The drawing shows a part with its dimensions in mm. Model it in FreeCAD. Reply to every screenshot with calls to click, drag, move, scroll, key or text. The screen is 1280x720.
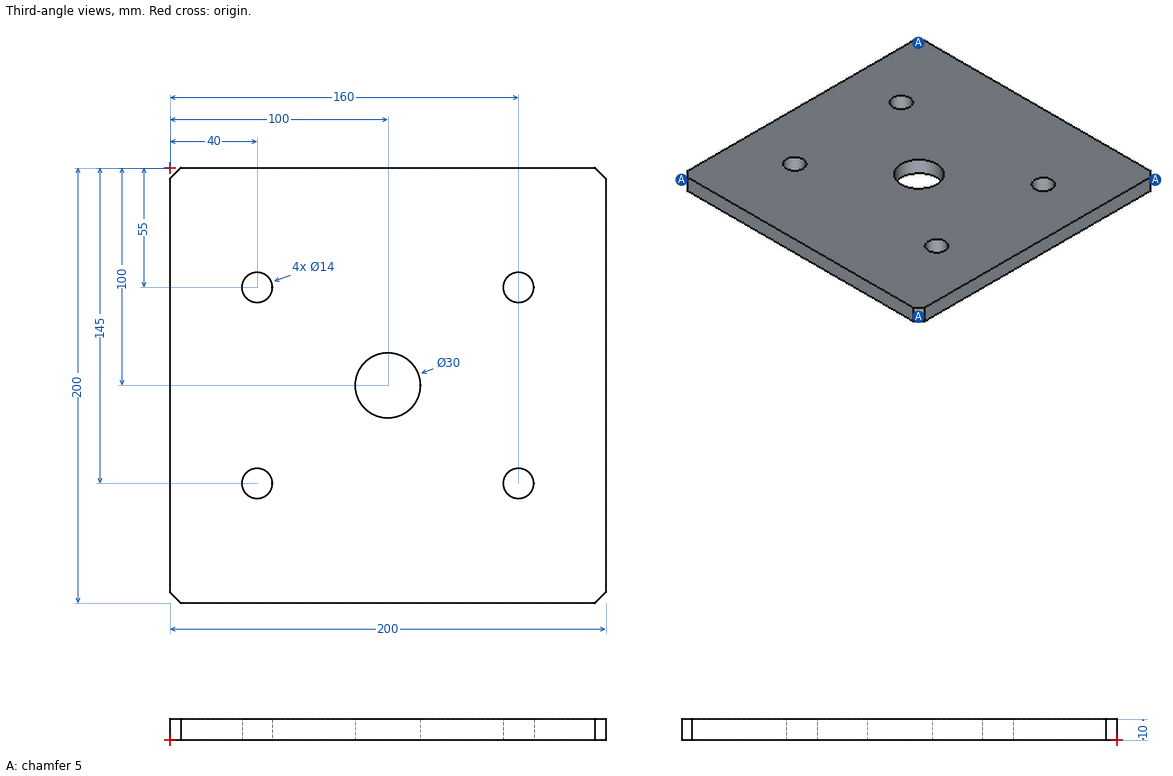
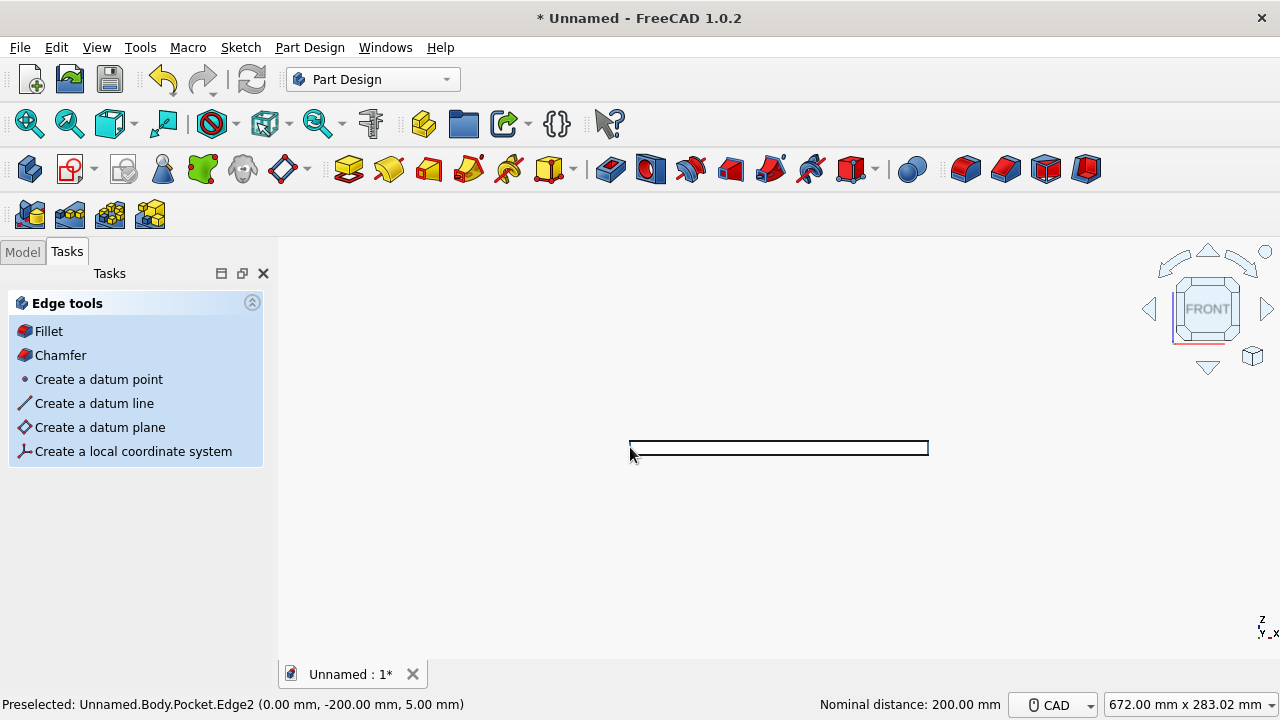
scroll(630, 447, up, 5)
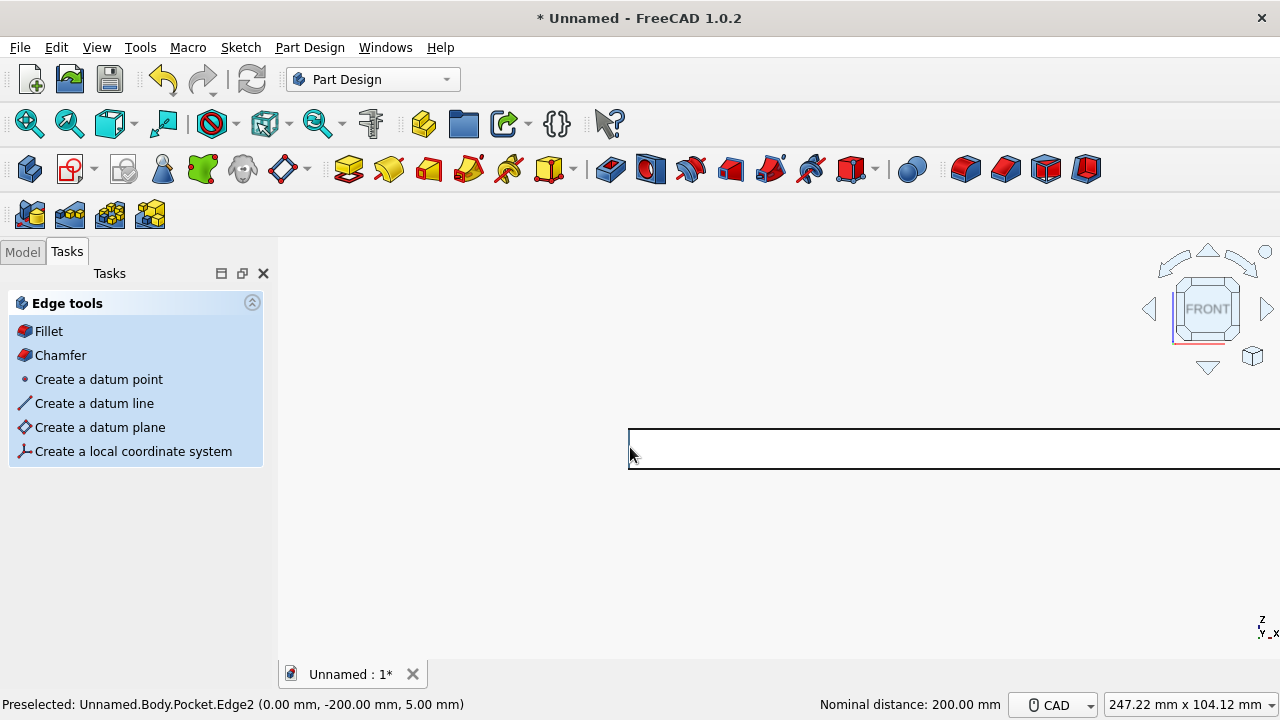
click(30, 124)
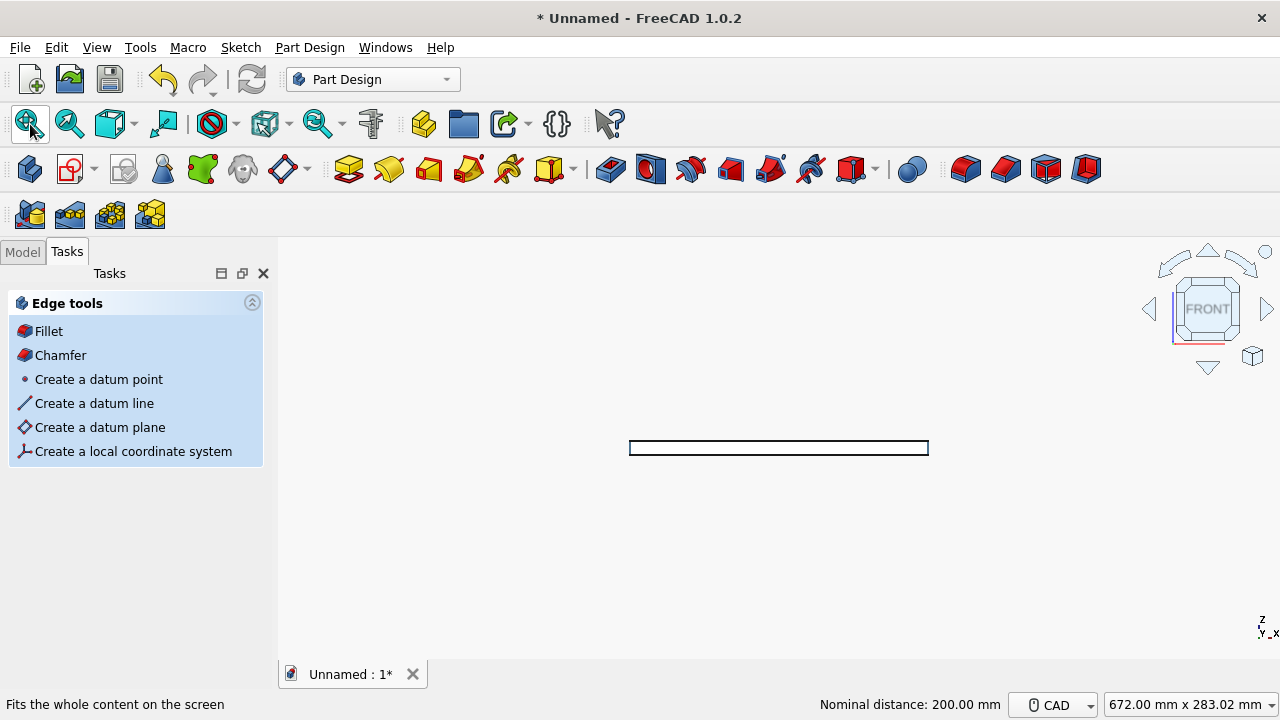
key(3)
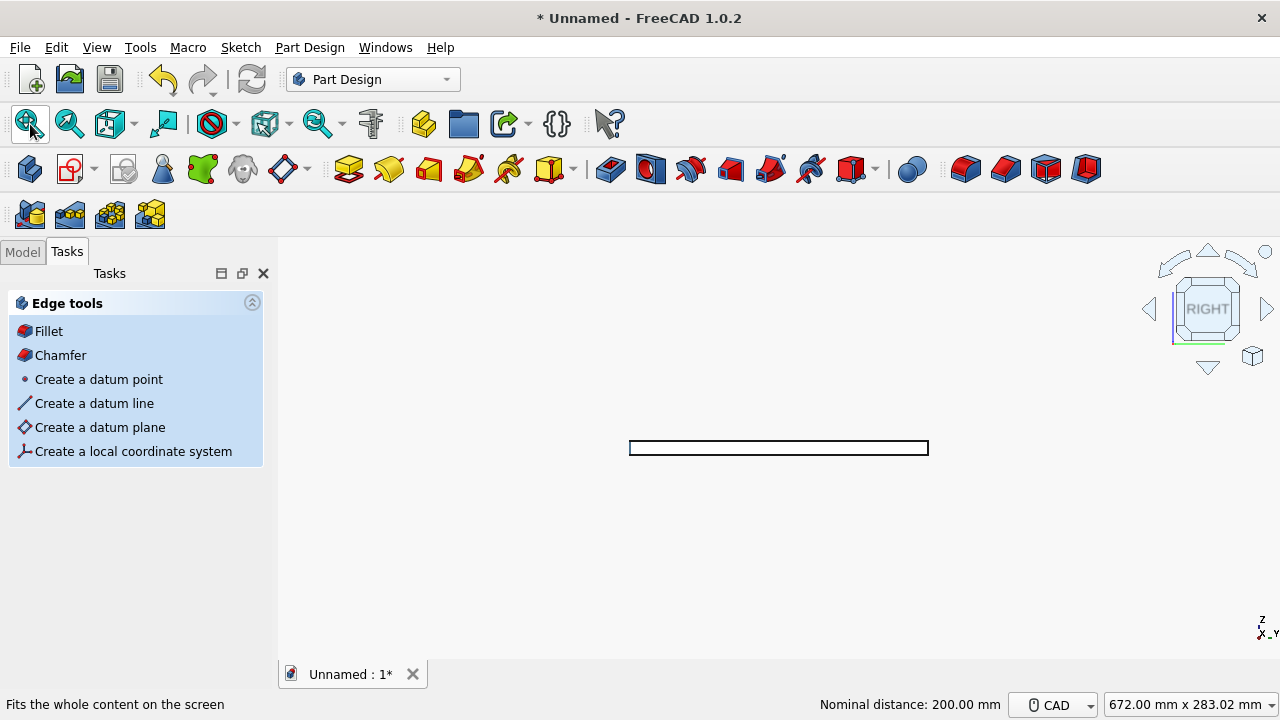
click(30, 124)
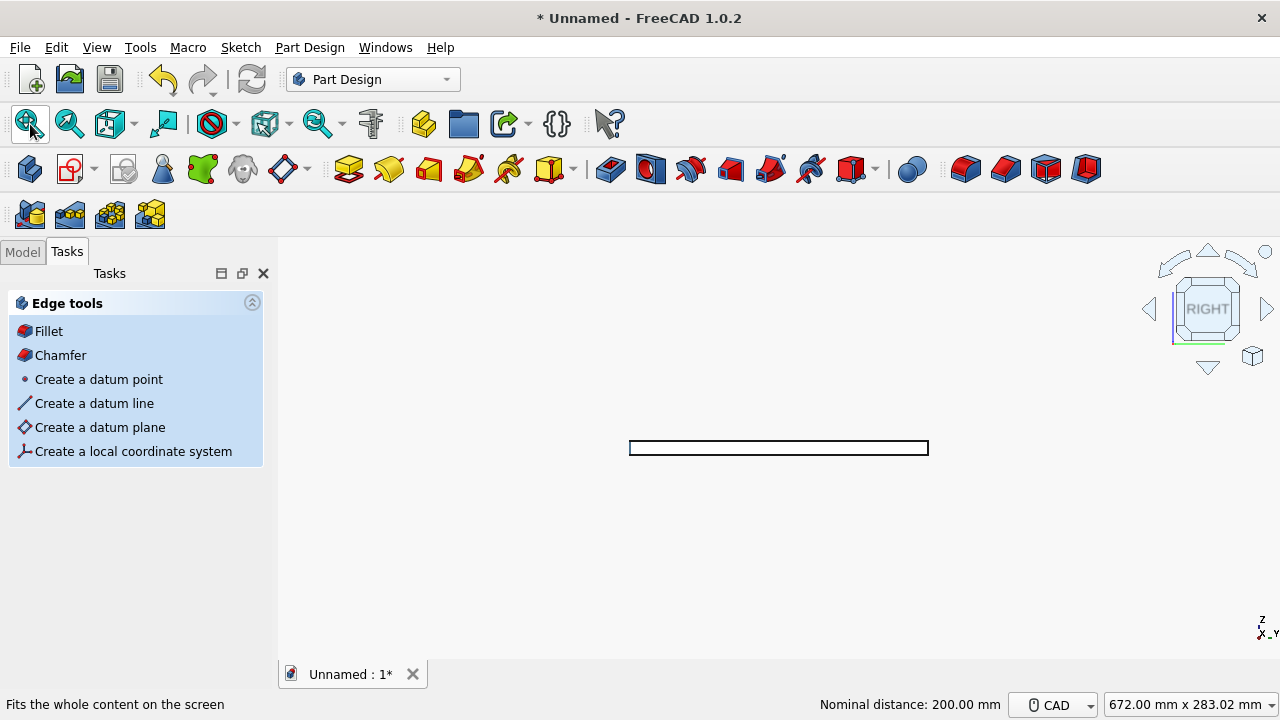
click(928, 447, ctrl)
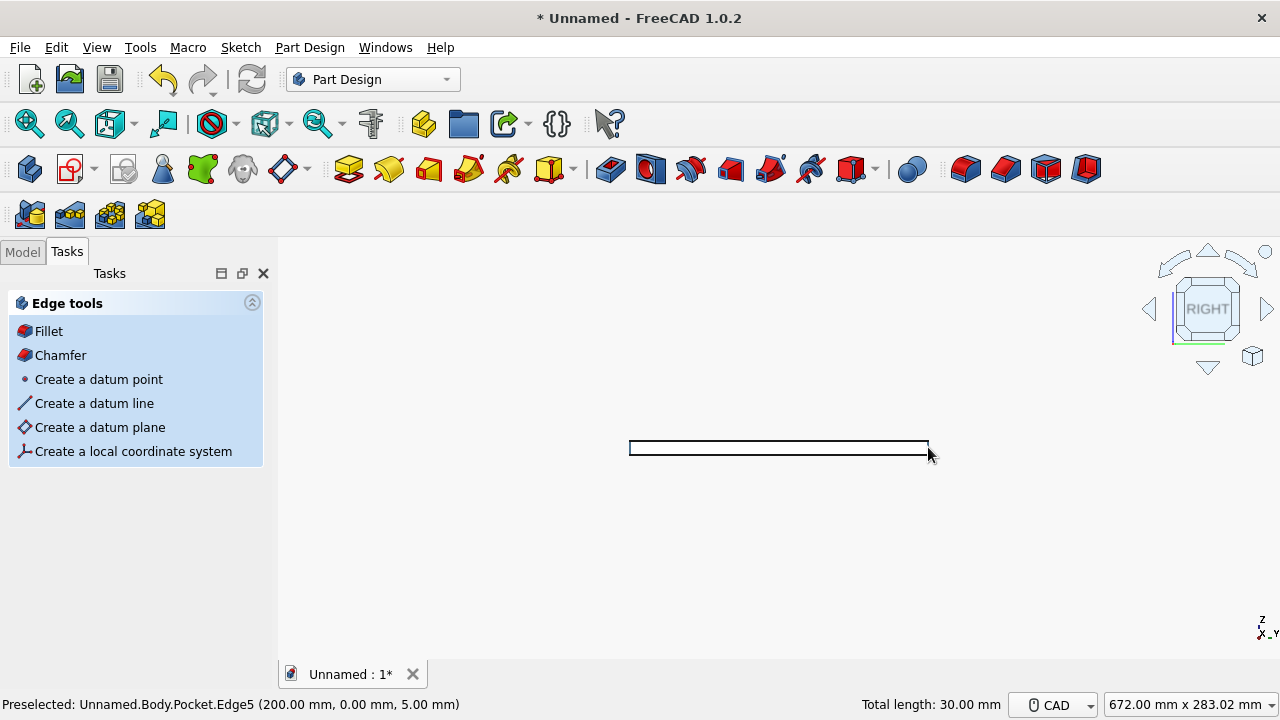
scroll(928, 447, up, 5)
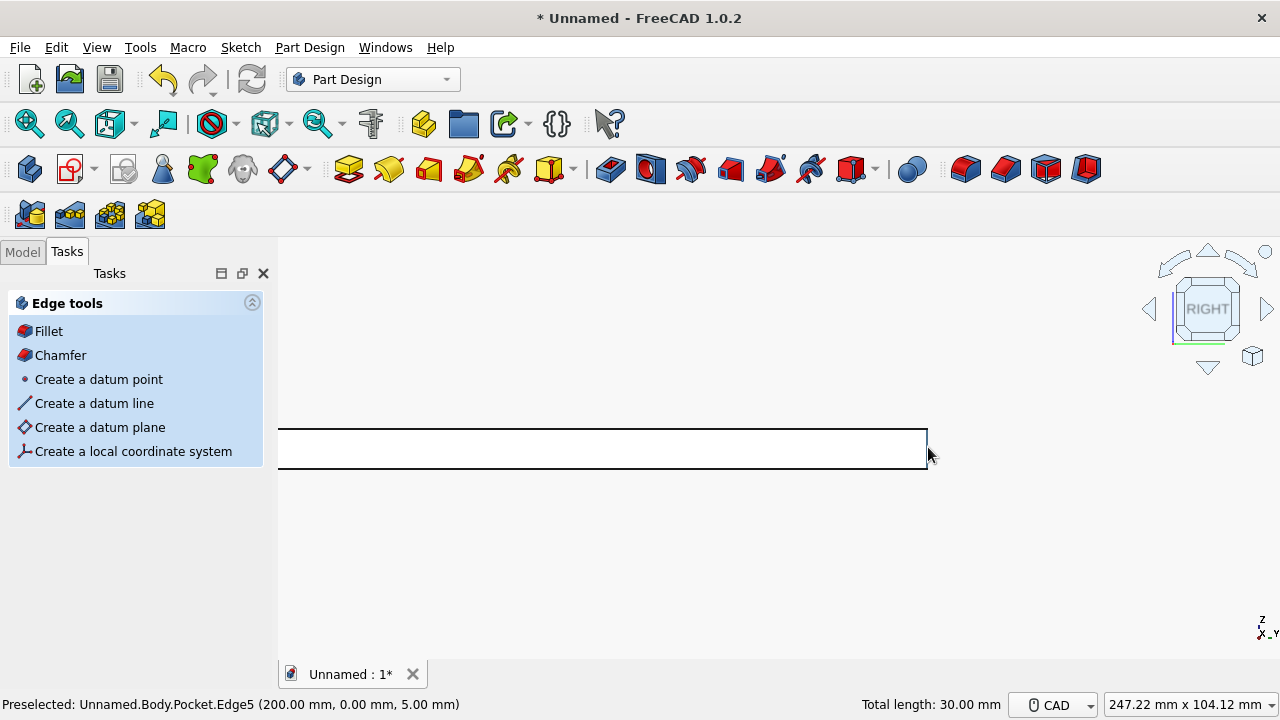
click(30, 124)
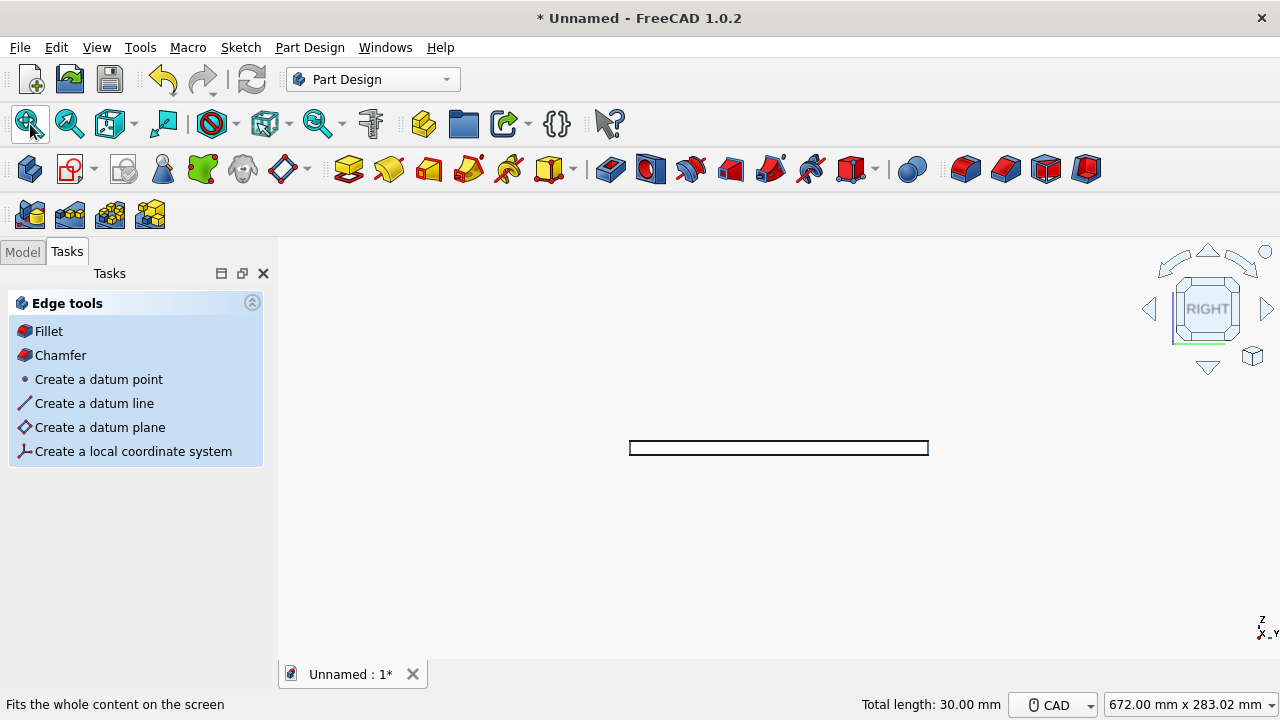
key(5)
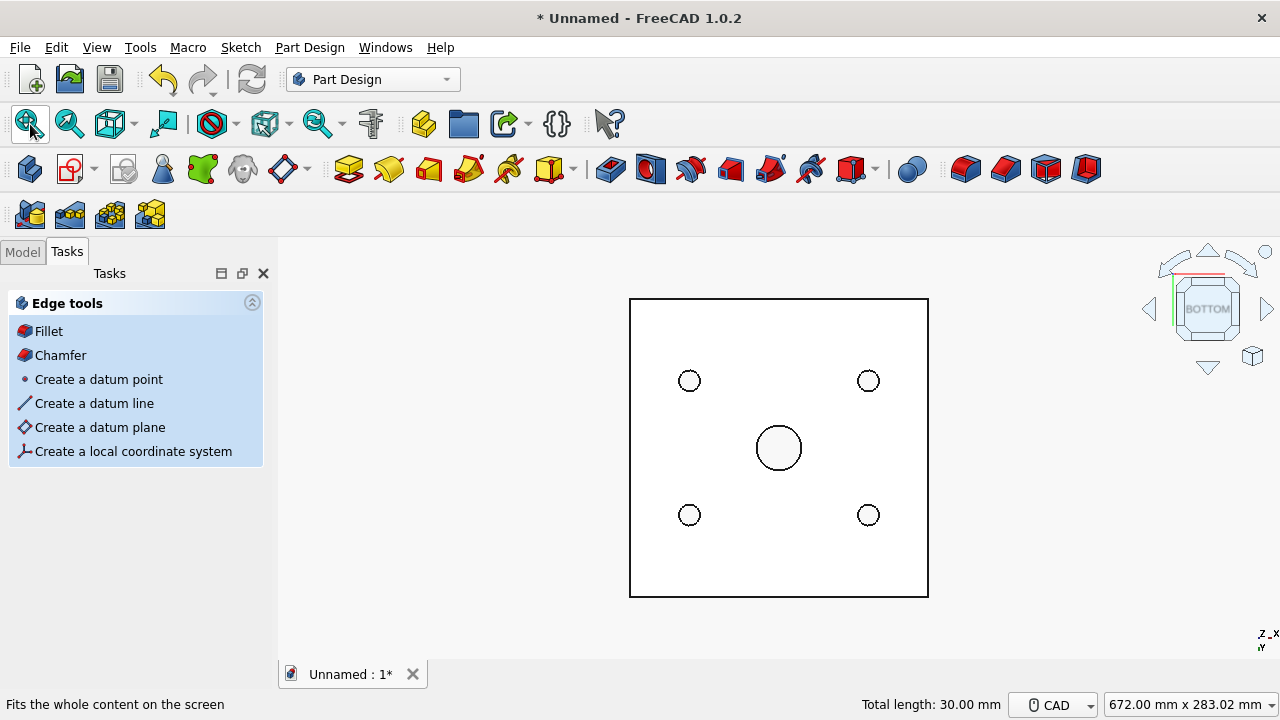
scroll(630, 596, up, 5)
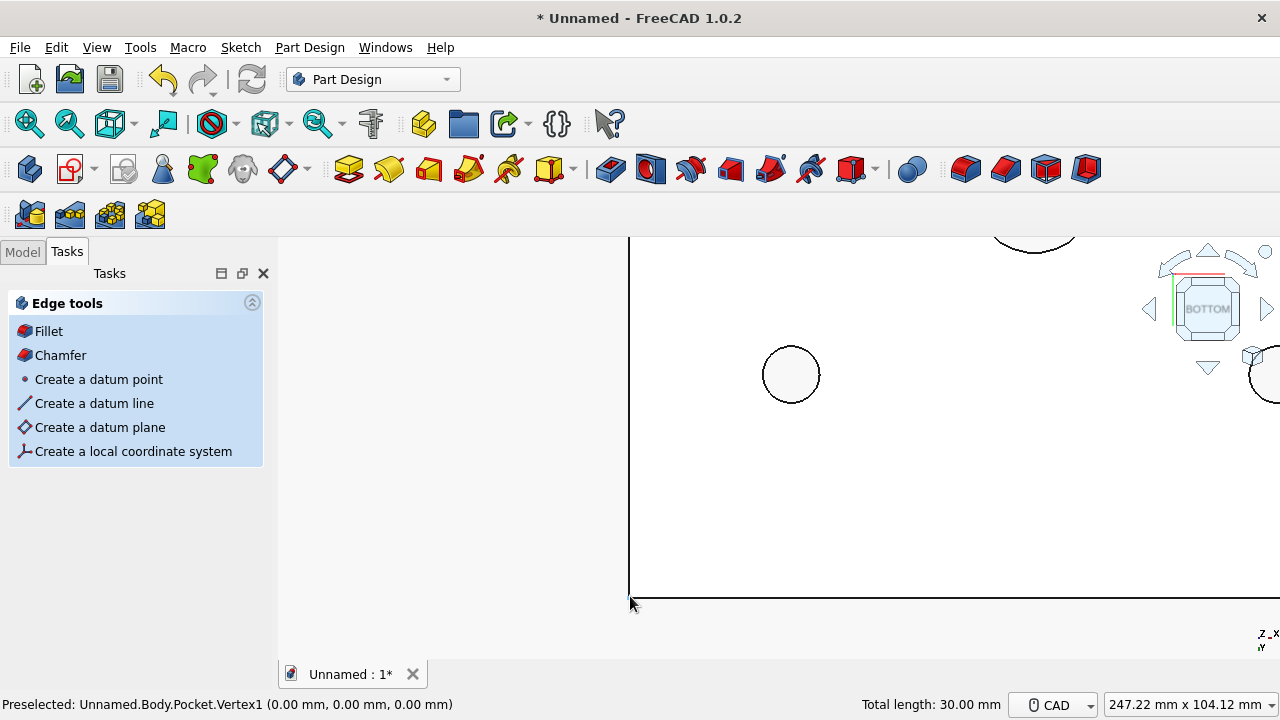
click(30, 124)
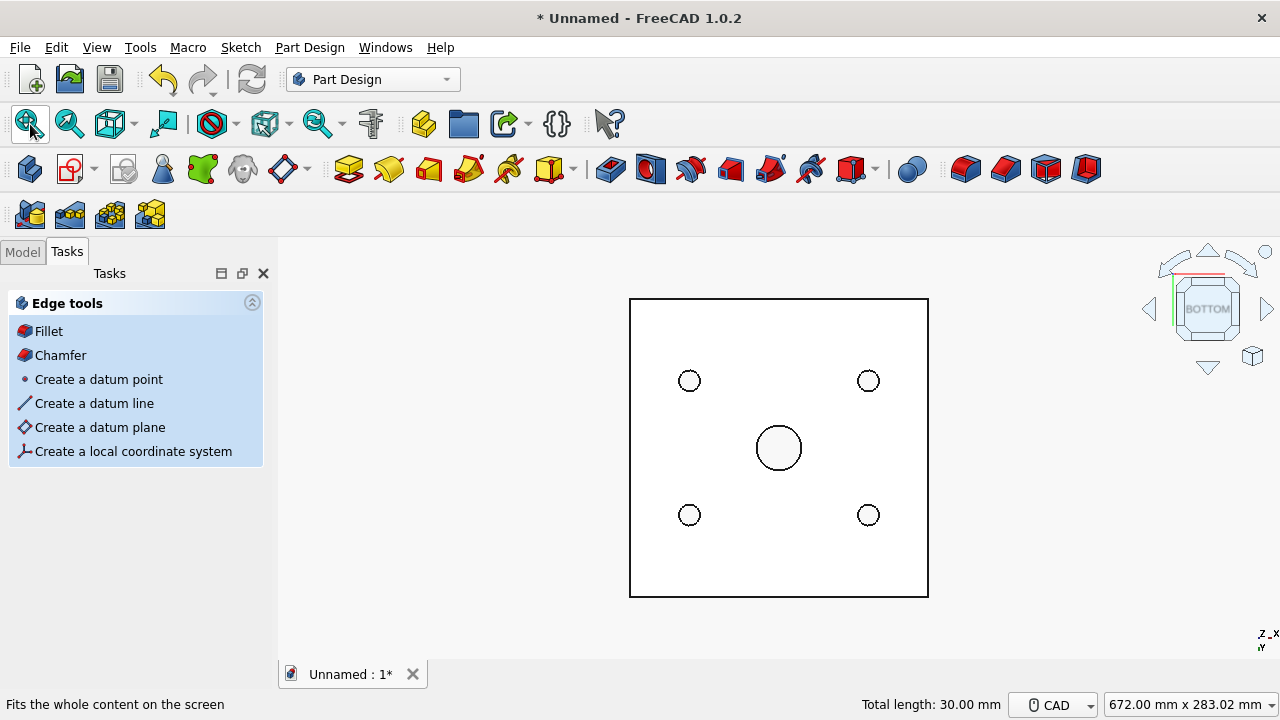
key(4)